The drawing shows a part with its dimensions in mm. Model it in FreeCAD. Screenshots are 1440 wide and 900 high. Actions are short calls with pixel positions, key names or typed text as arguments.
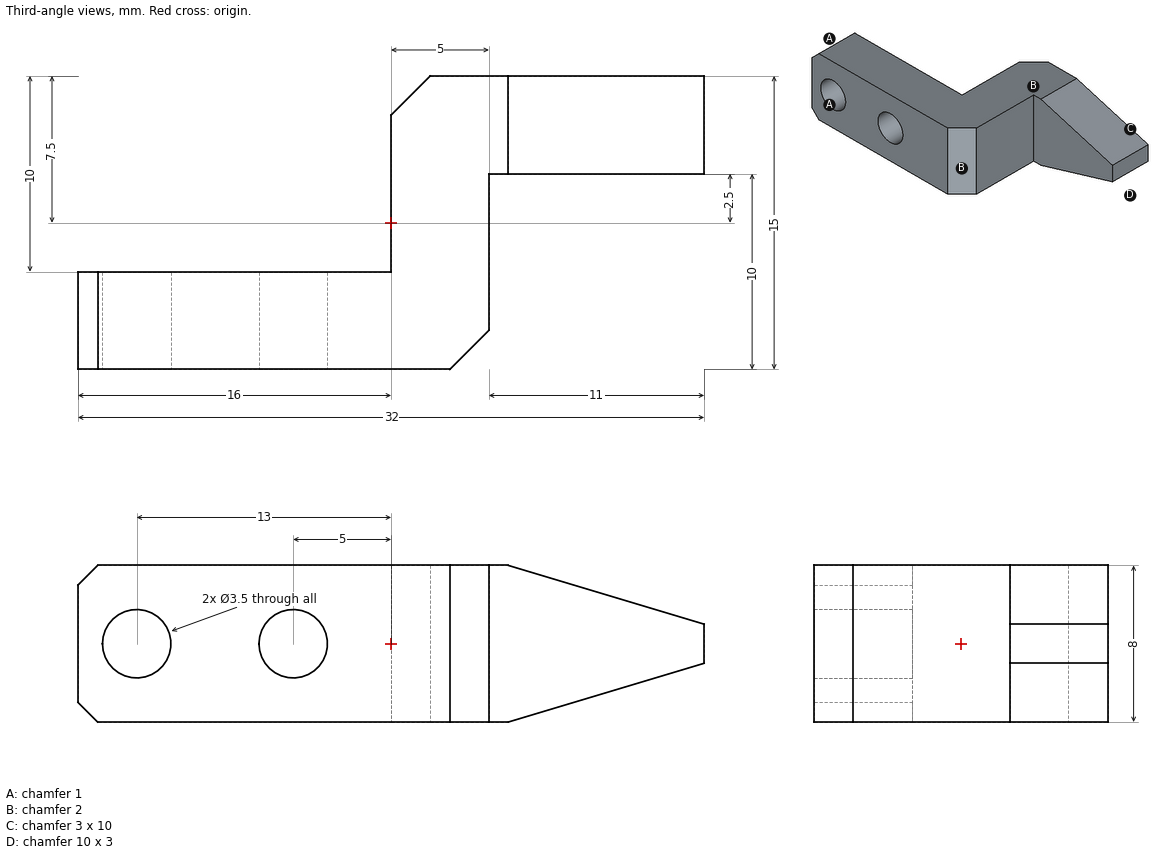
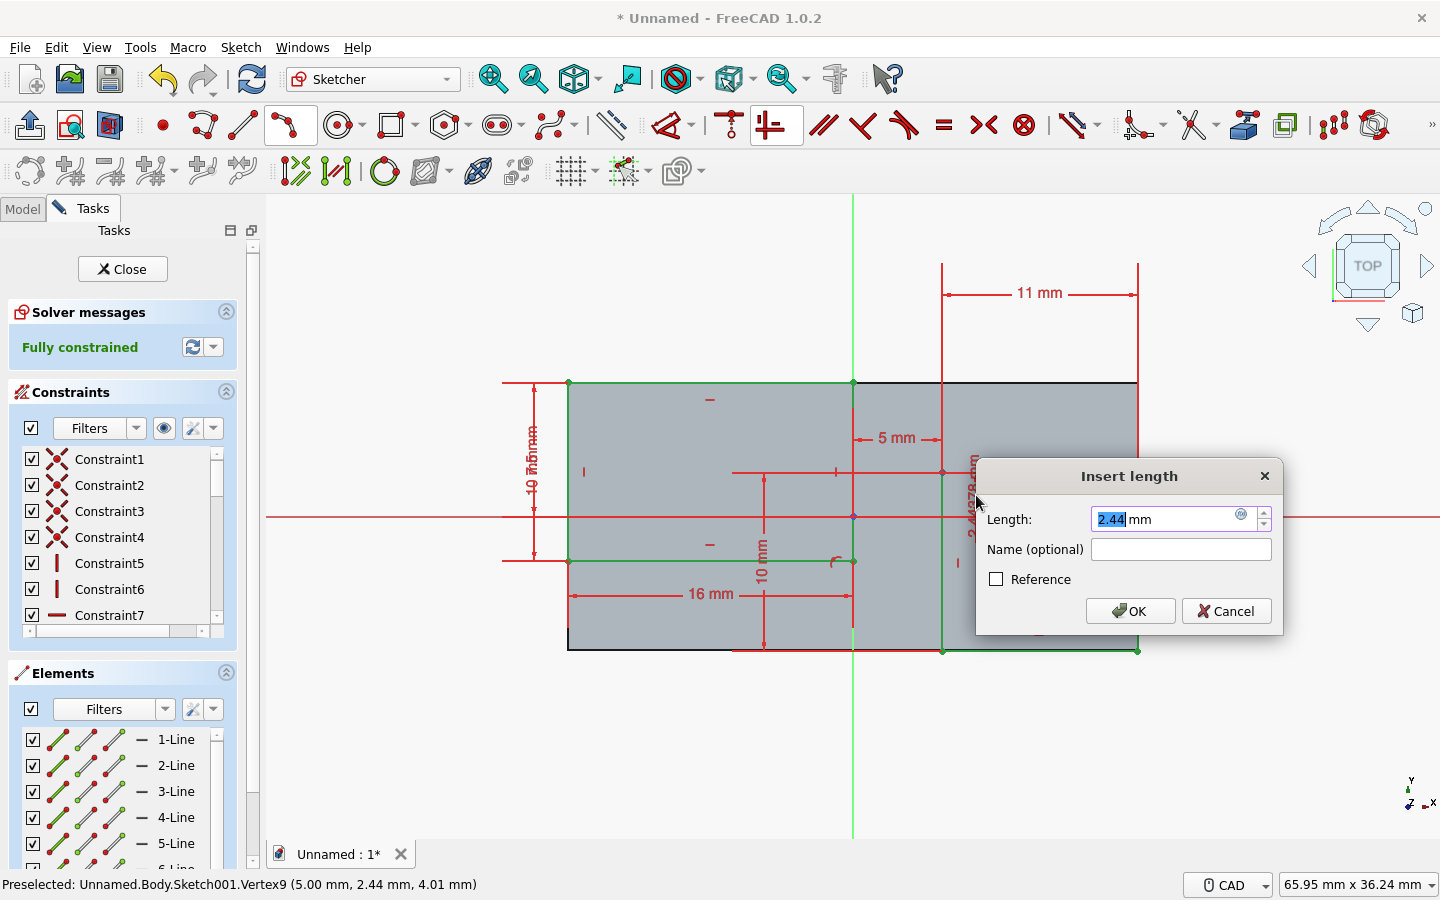
text(2.5)
key(Return)
key(Escape)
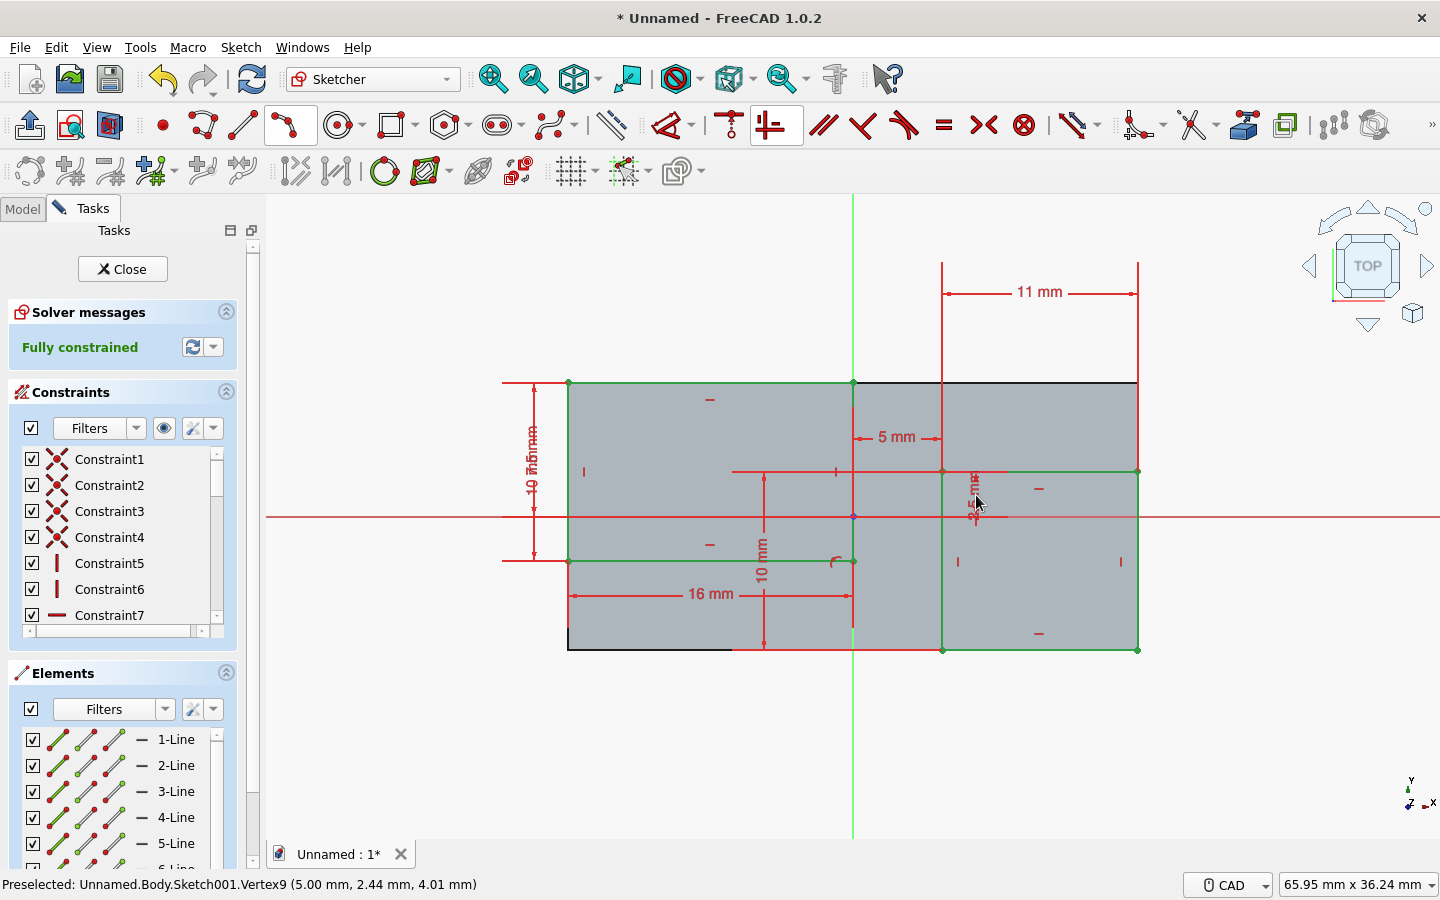
click(123, 269)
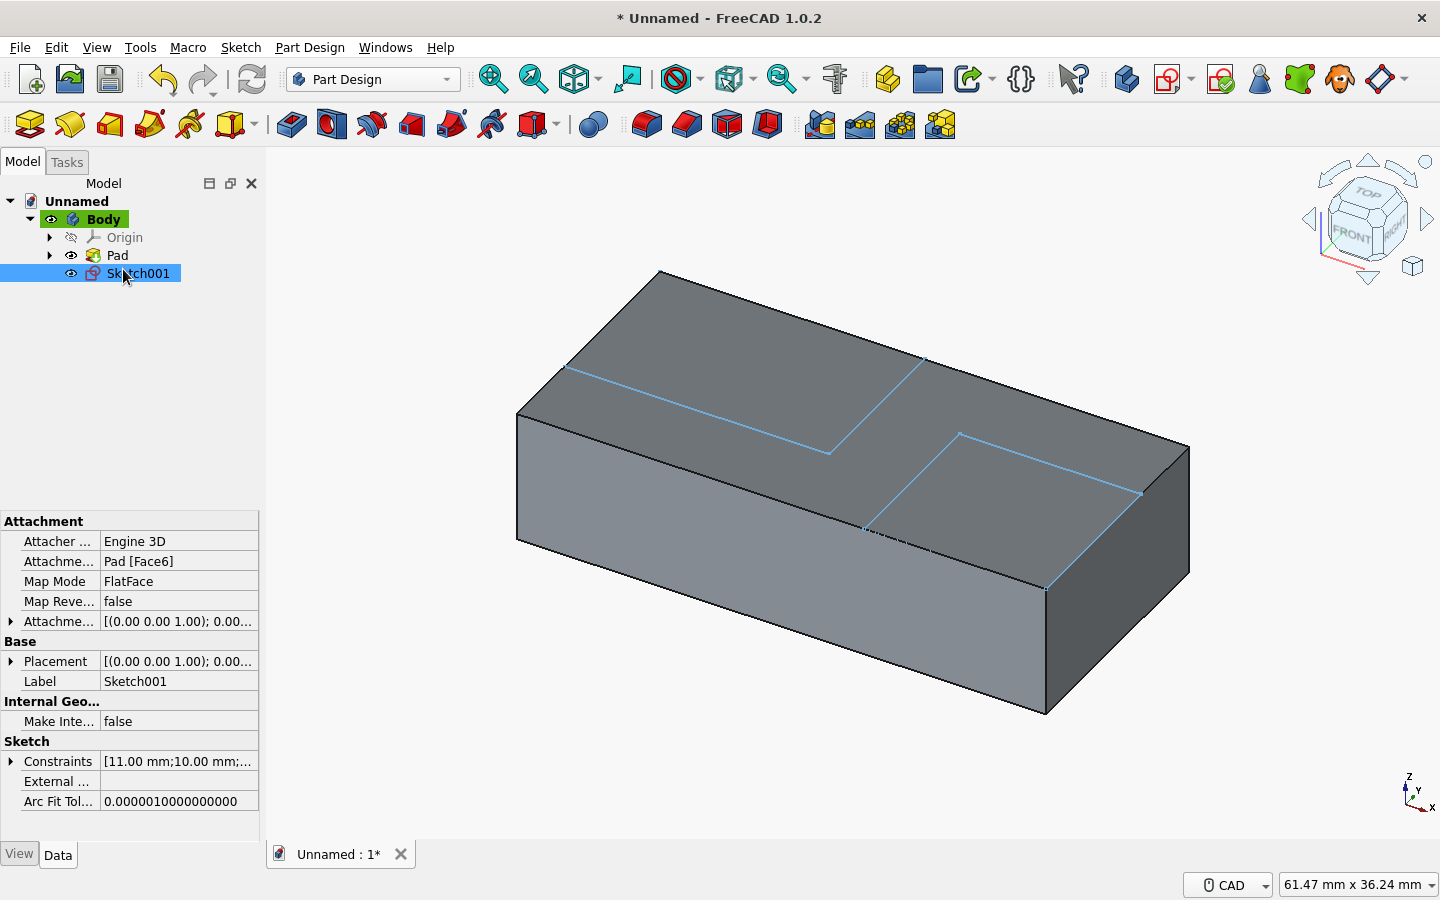
click(292, 124)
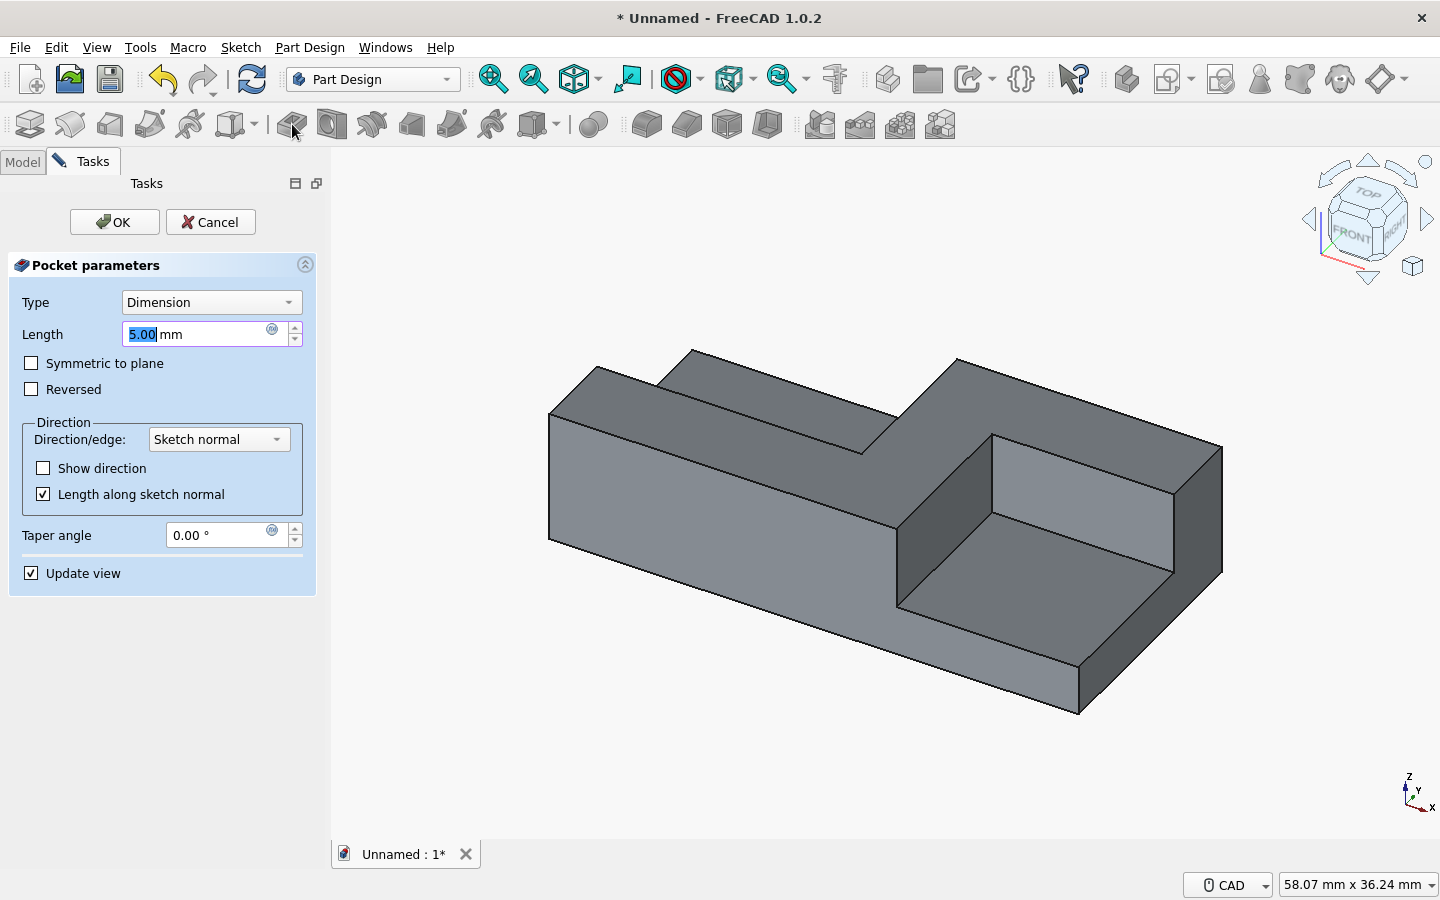
click(212, 302)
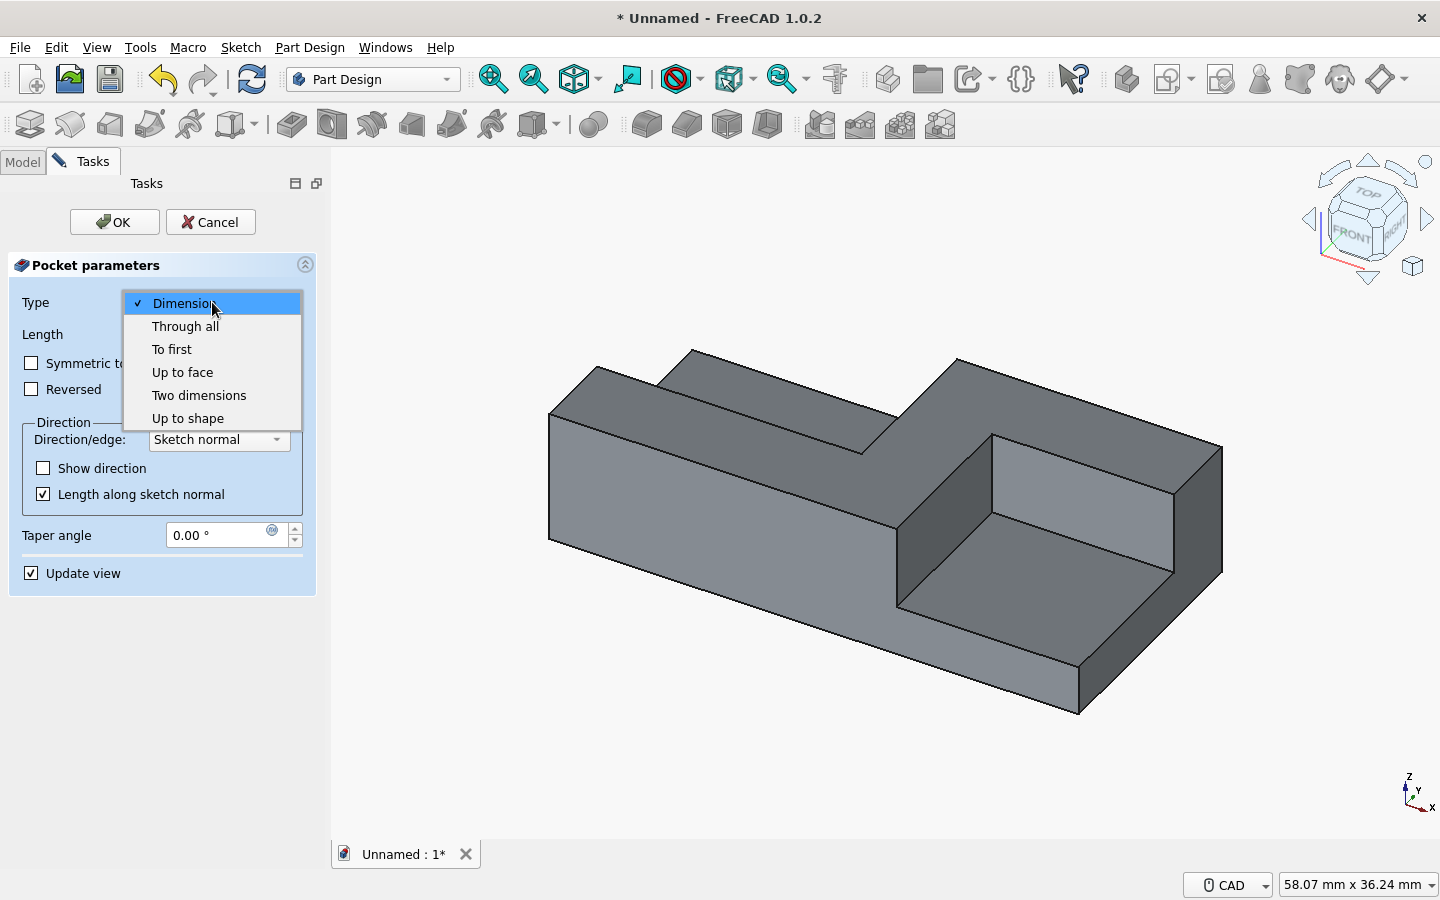
click(212, 326)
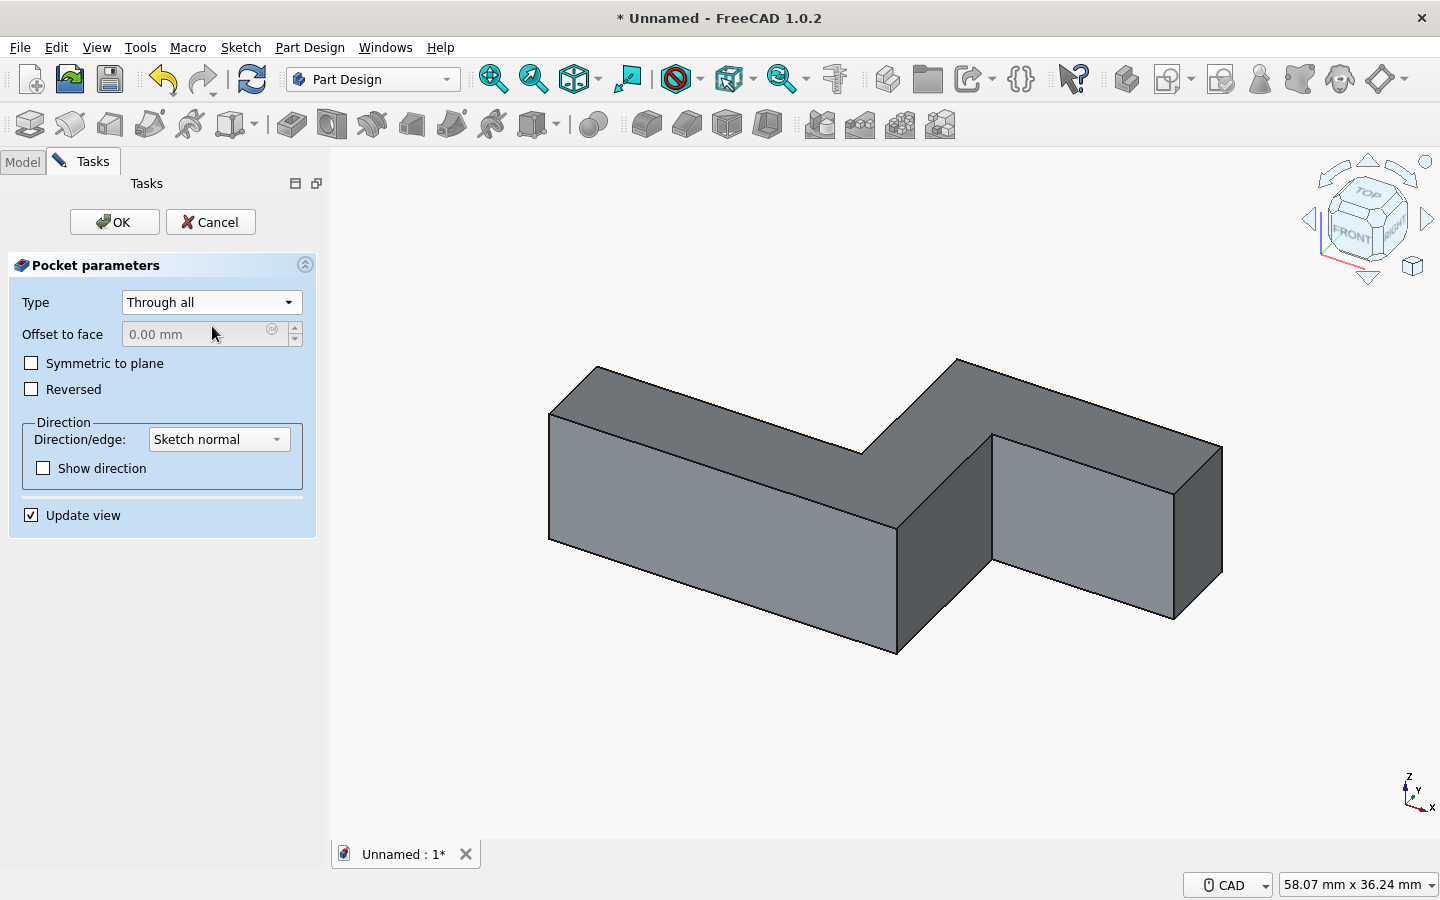
click(115, 222)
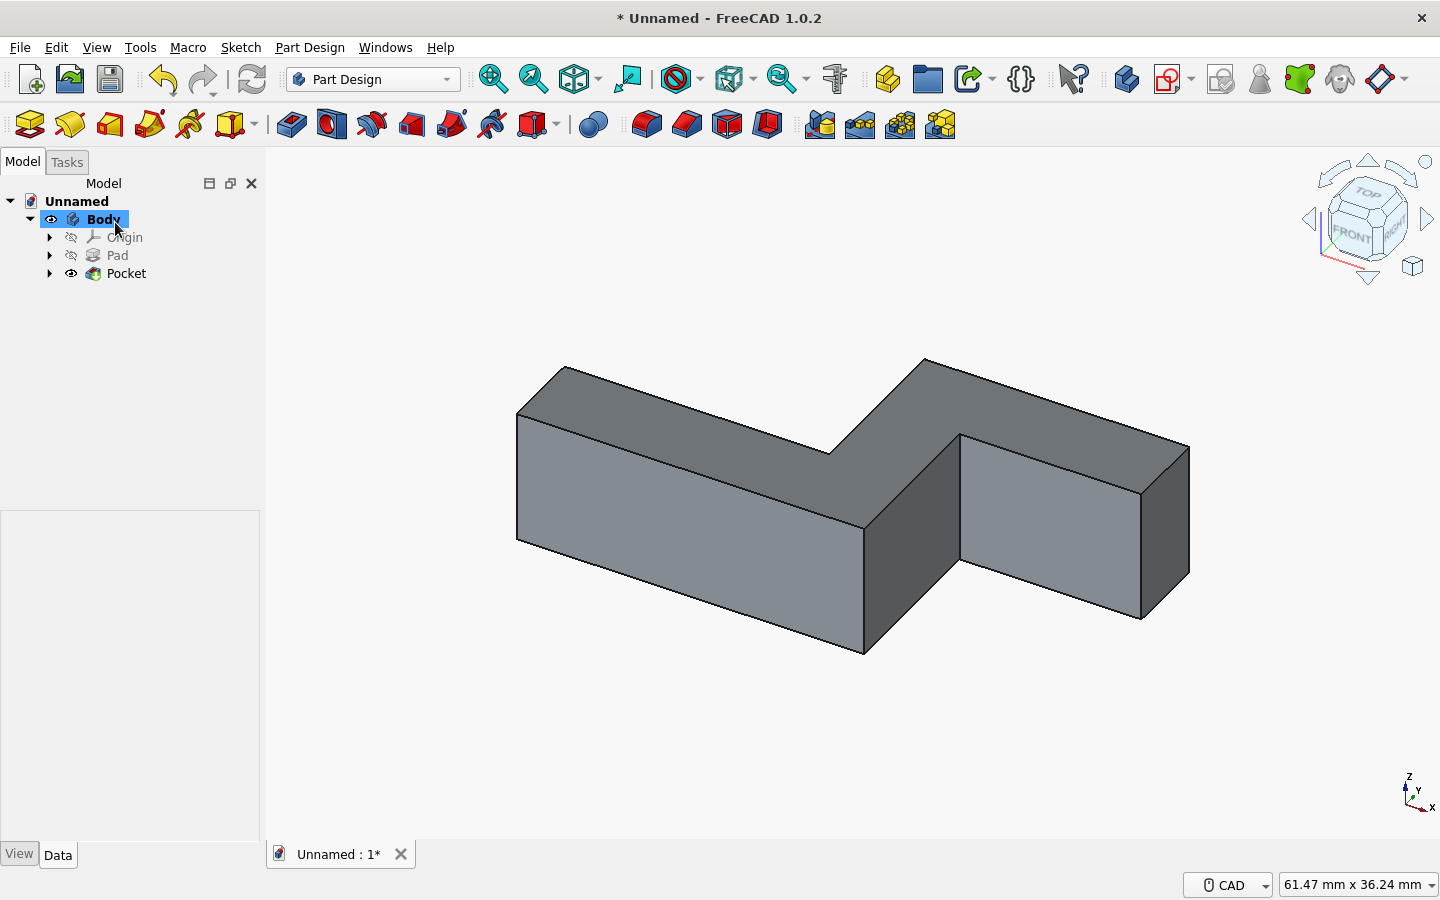
key(0)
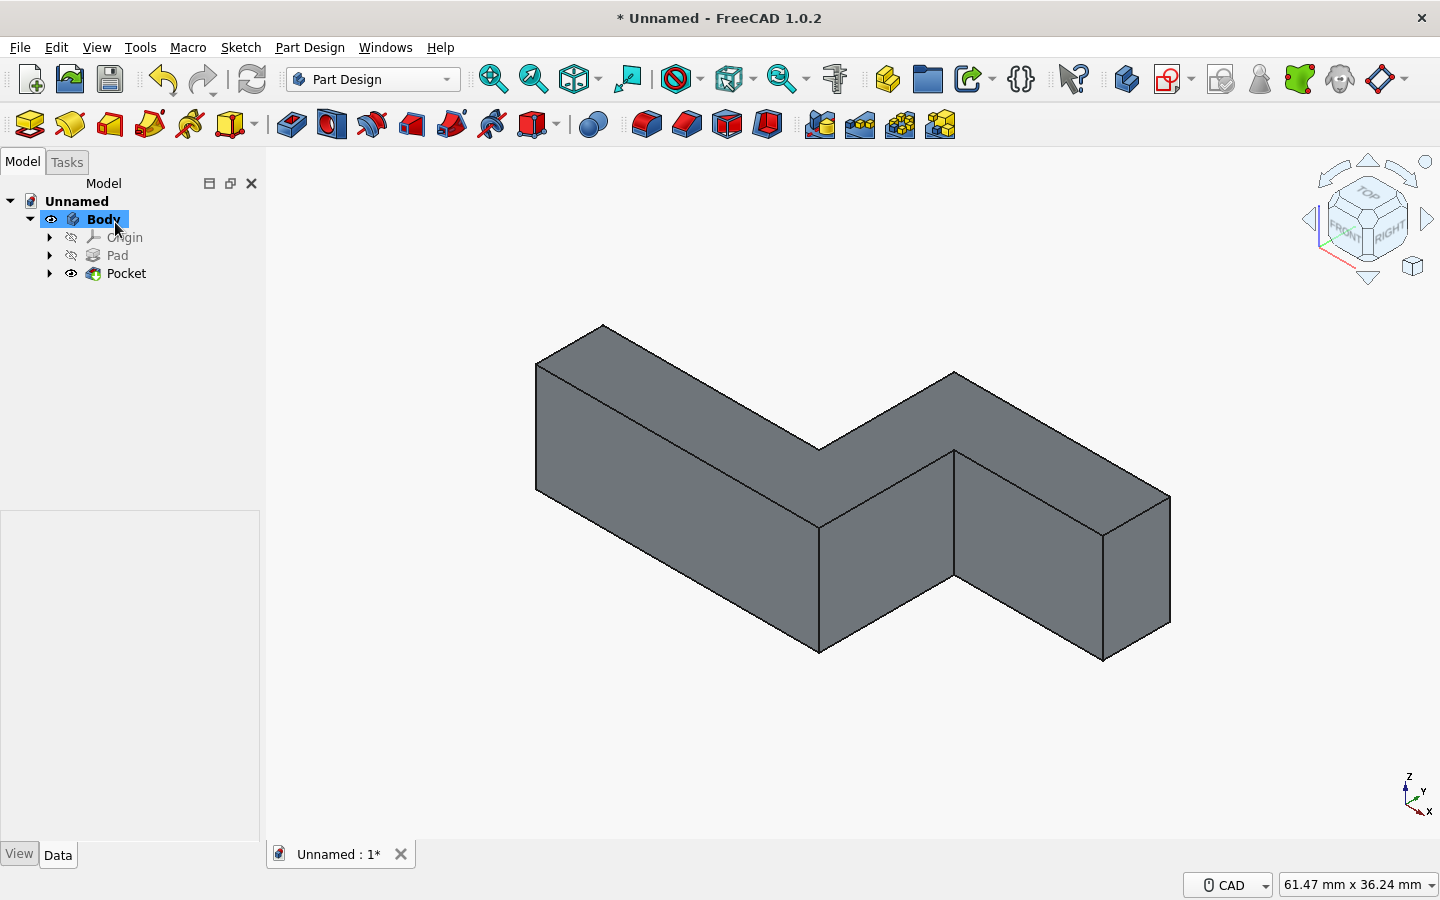
key(2)